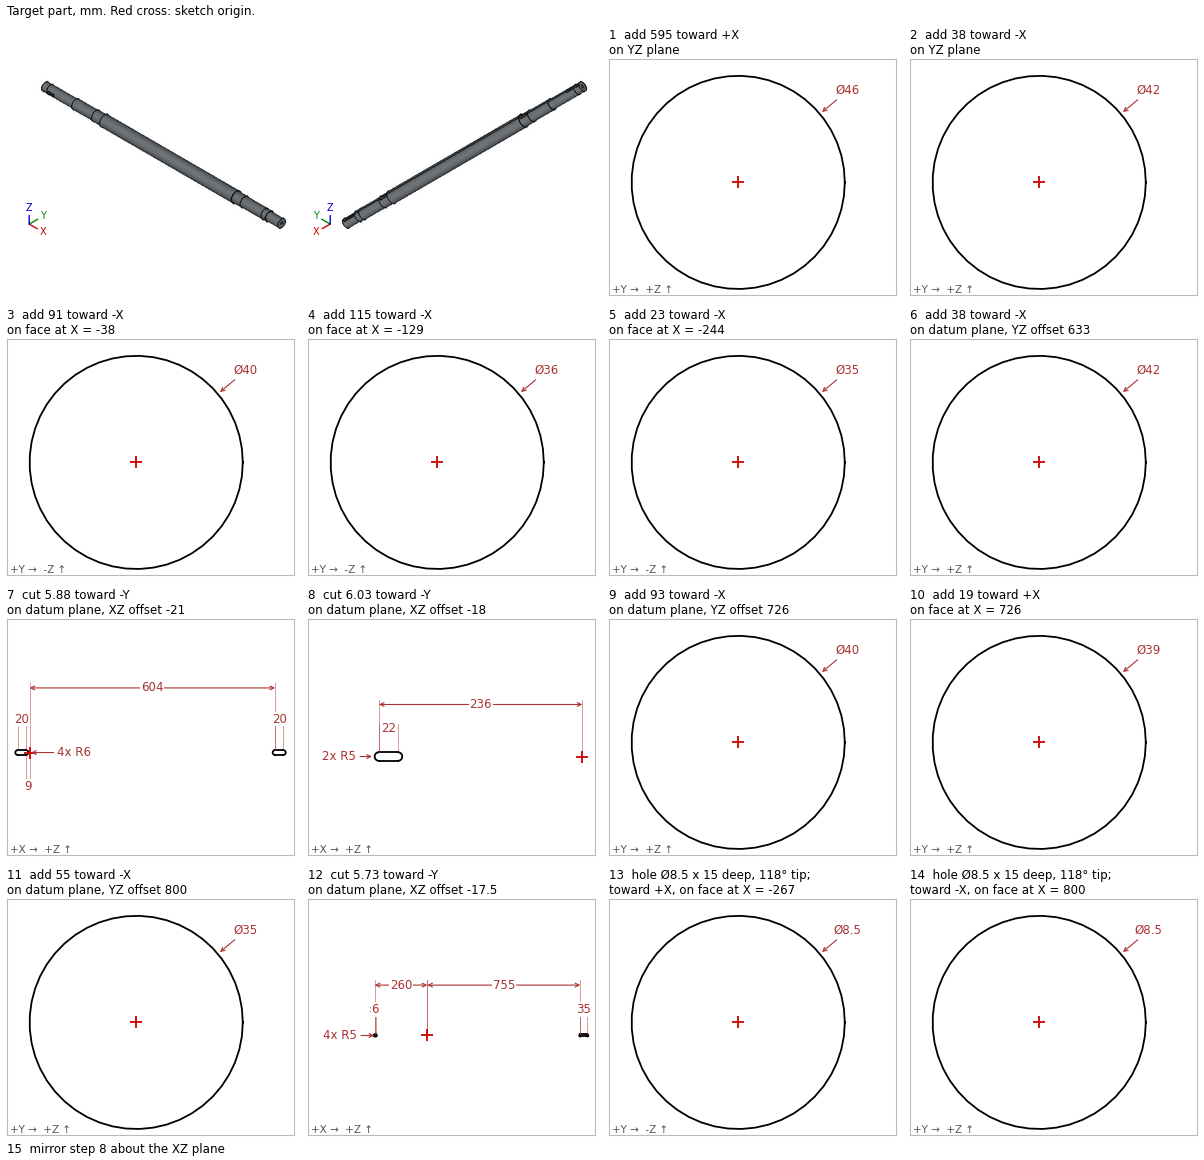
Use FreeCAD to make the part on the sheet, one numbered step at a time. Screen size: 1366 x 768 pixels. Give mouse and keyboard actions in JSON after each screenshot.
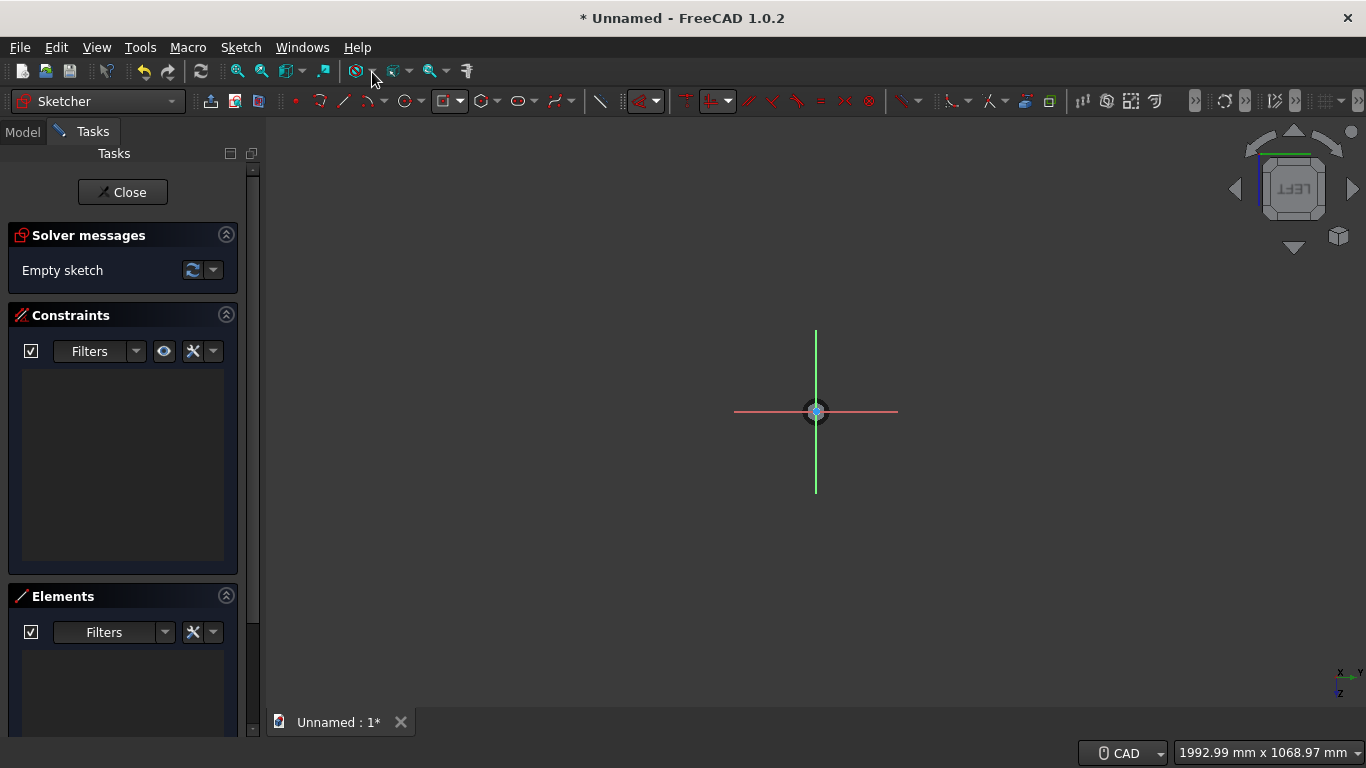
{"action": "scroll", "coordinate": [820, 412], "scroll_direction": "up", "scroll_amount": 15}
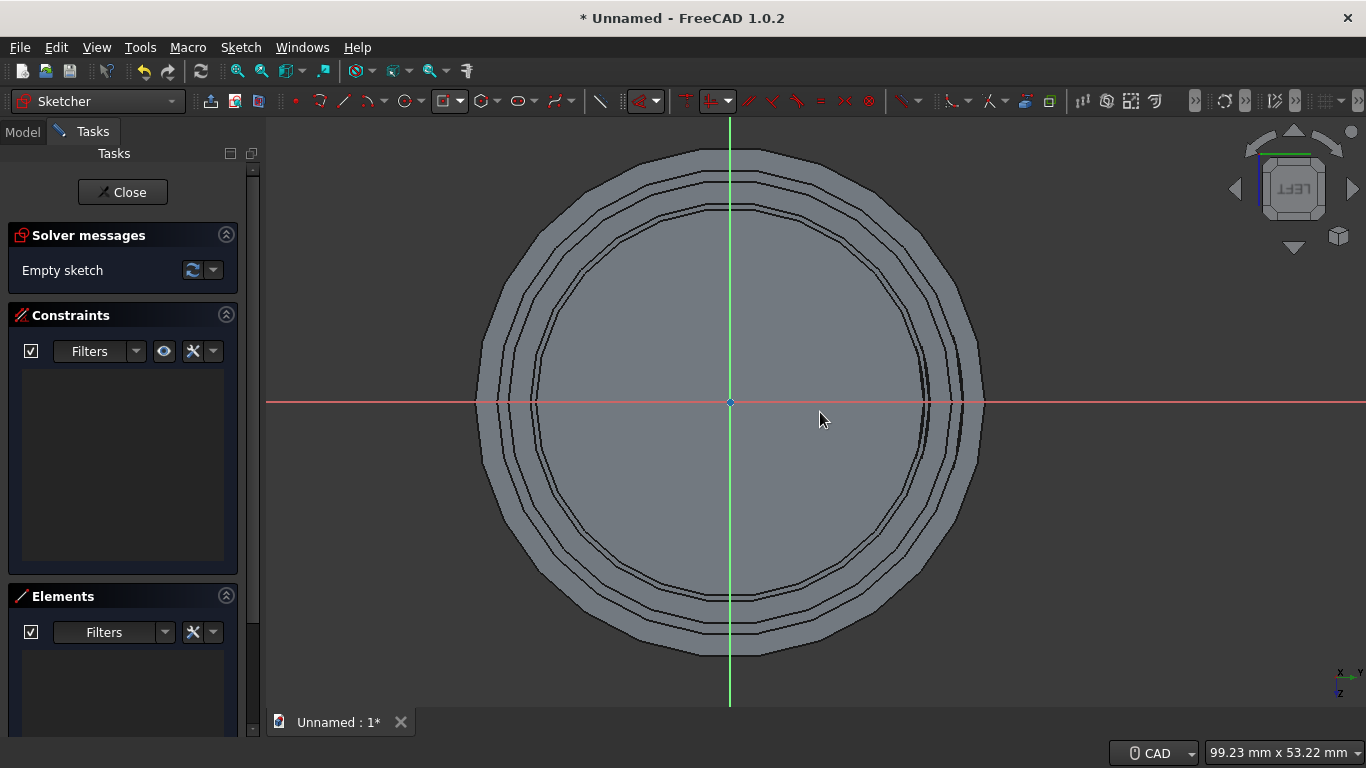
{"action": "scroll", "coordinate": [724, 399], "scroll_direction": "up", "scroll_amount": 7}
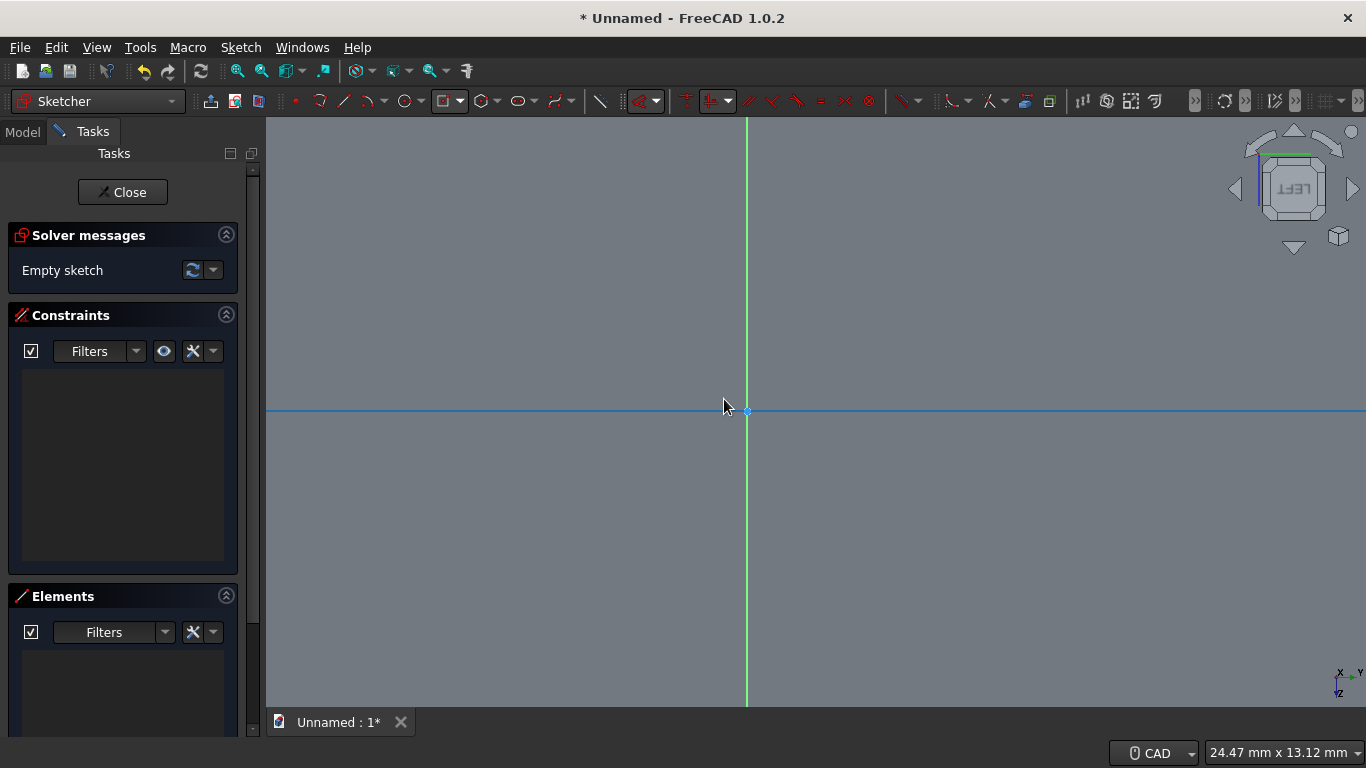
{"action": "key", "text": "g c"}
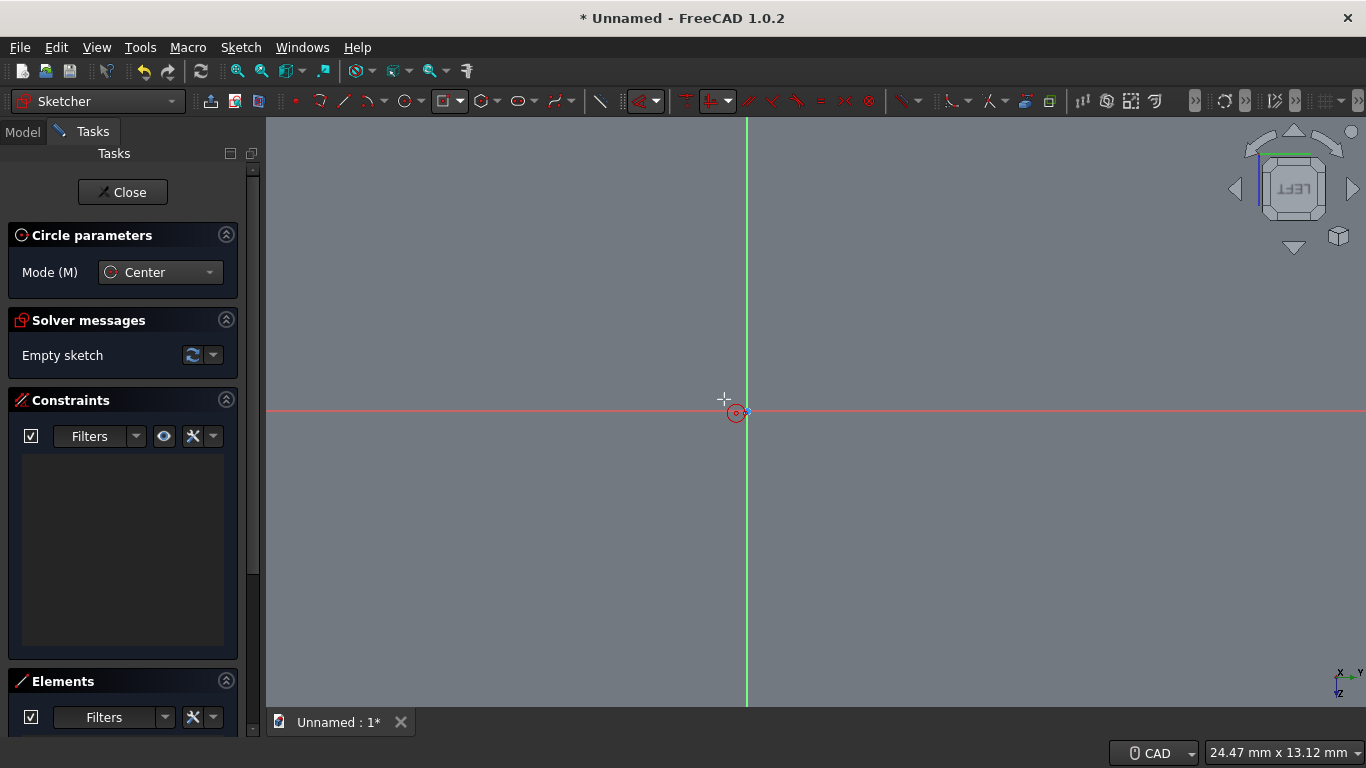
{"action": "left_click", "coordinate": [747, 411]}
{"action": "mouse_move", "coordinate": [882, 276]}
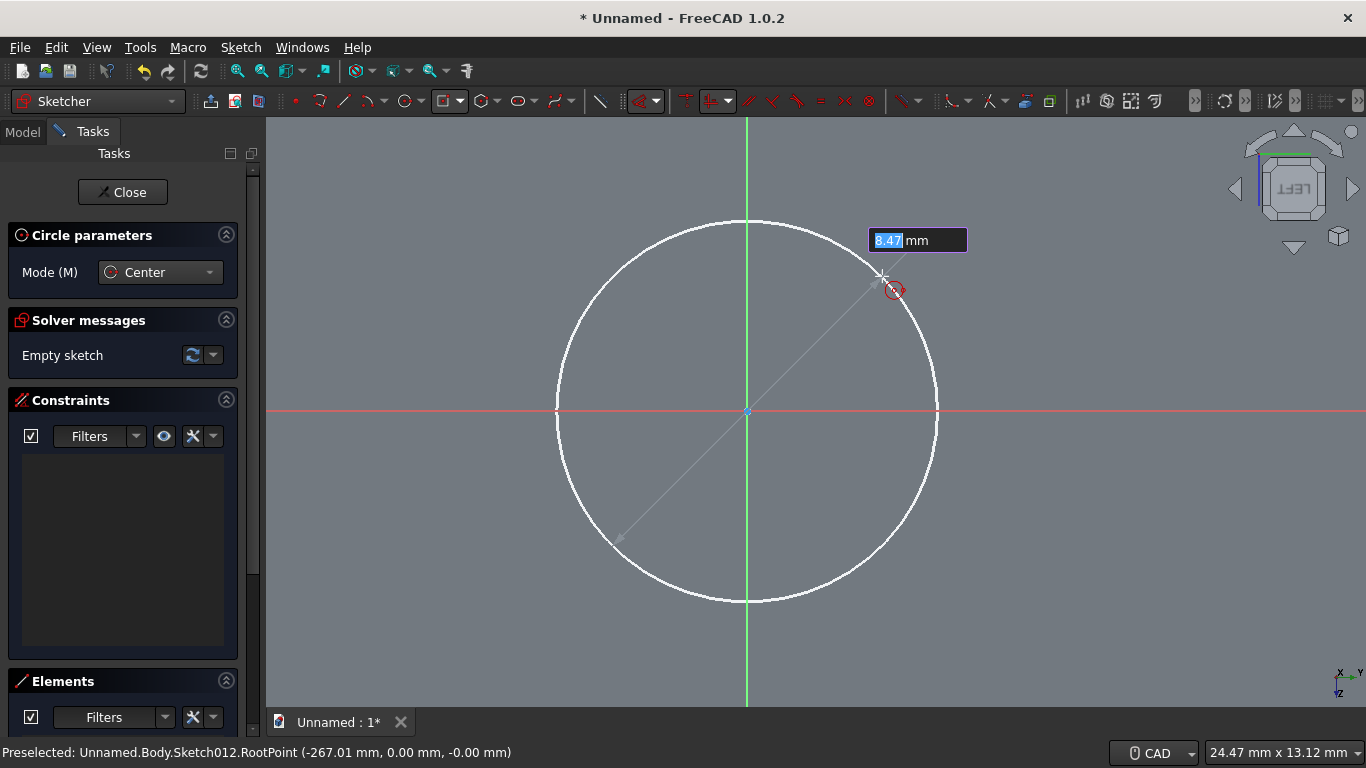
{"action": "type", "text": "8.5"}
{"action": "key", "text": "Return"}
{"action": "key", "text": "Escape"}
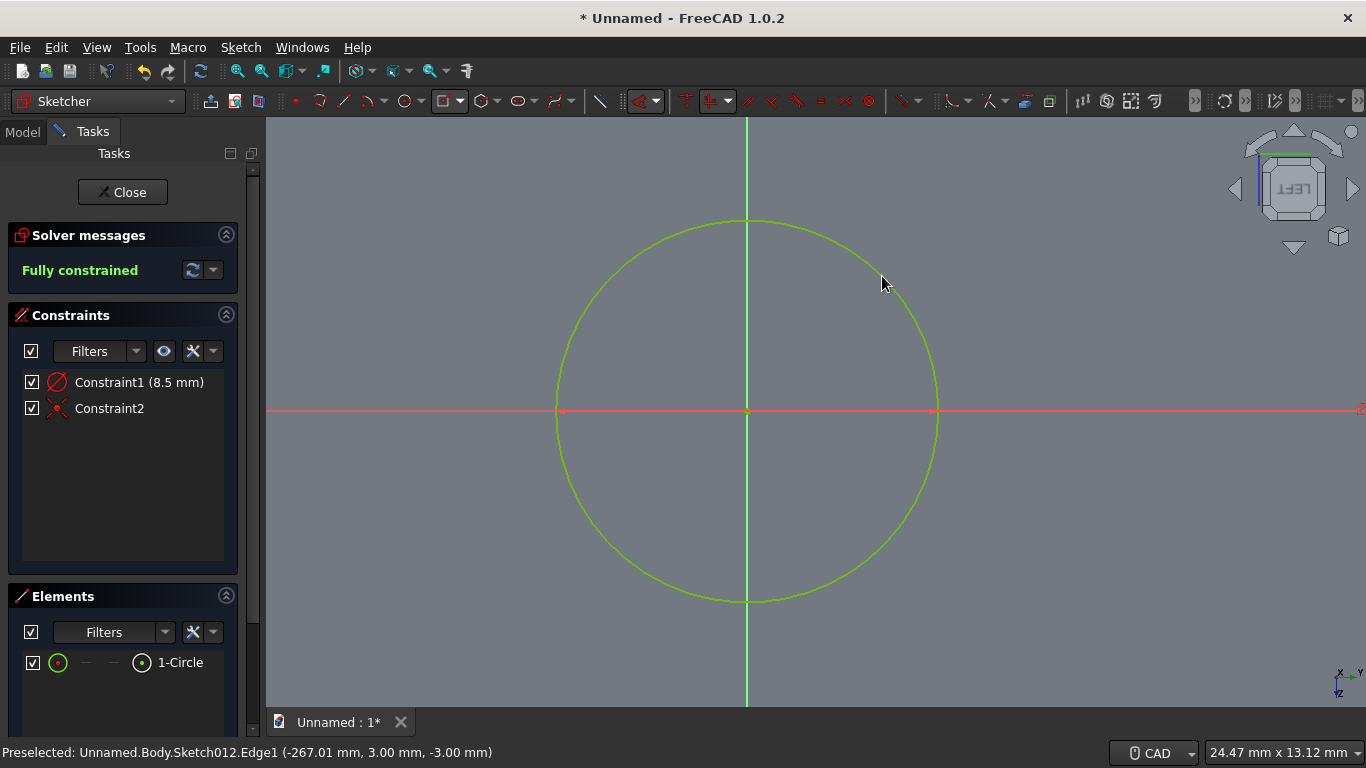
{"action": "left_click", "coordinate": [123, 192]}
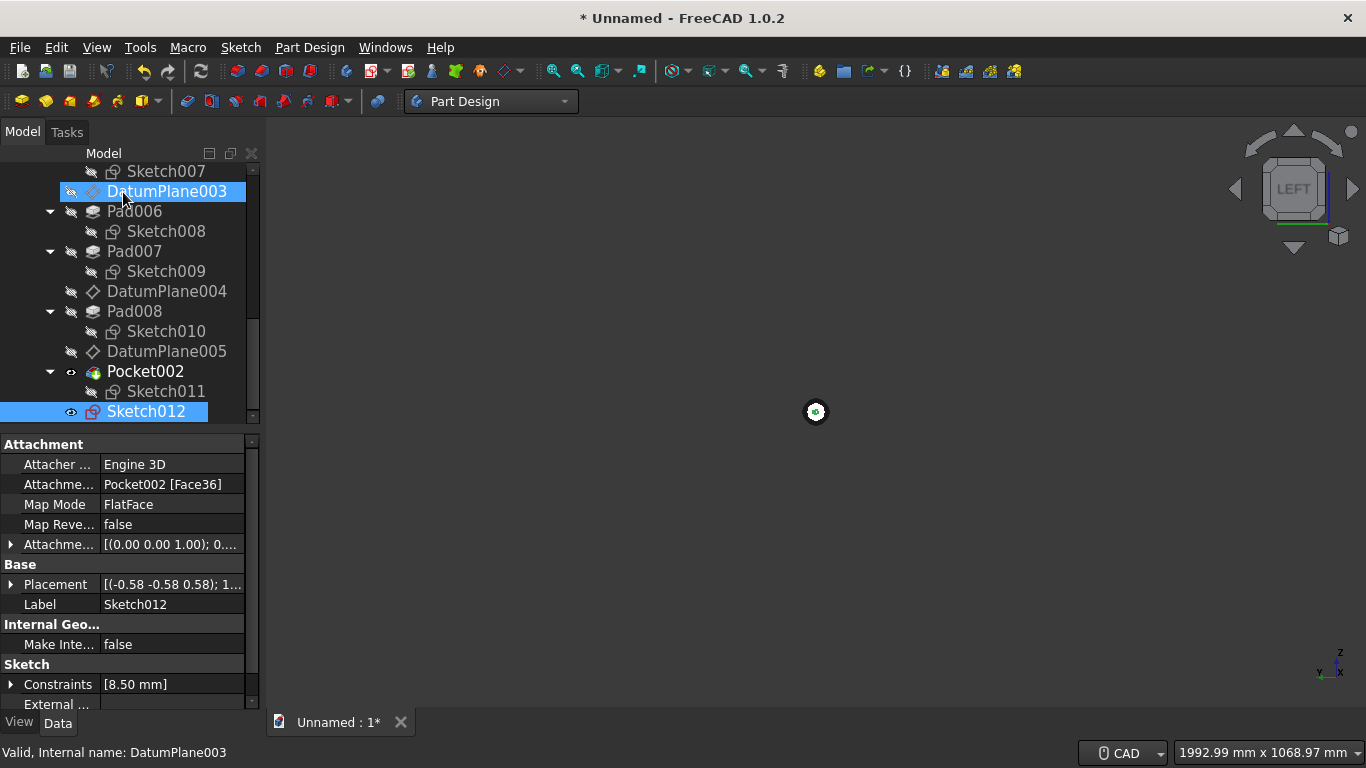
{"action": "left_click", "coordinate": [212, 102]}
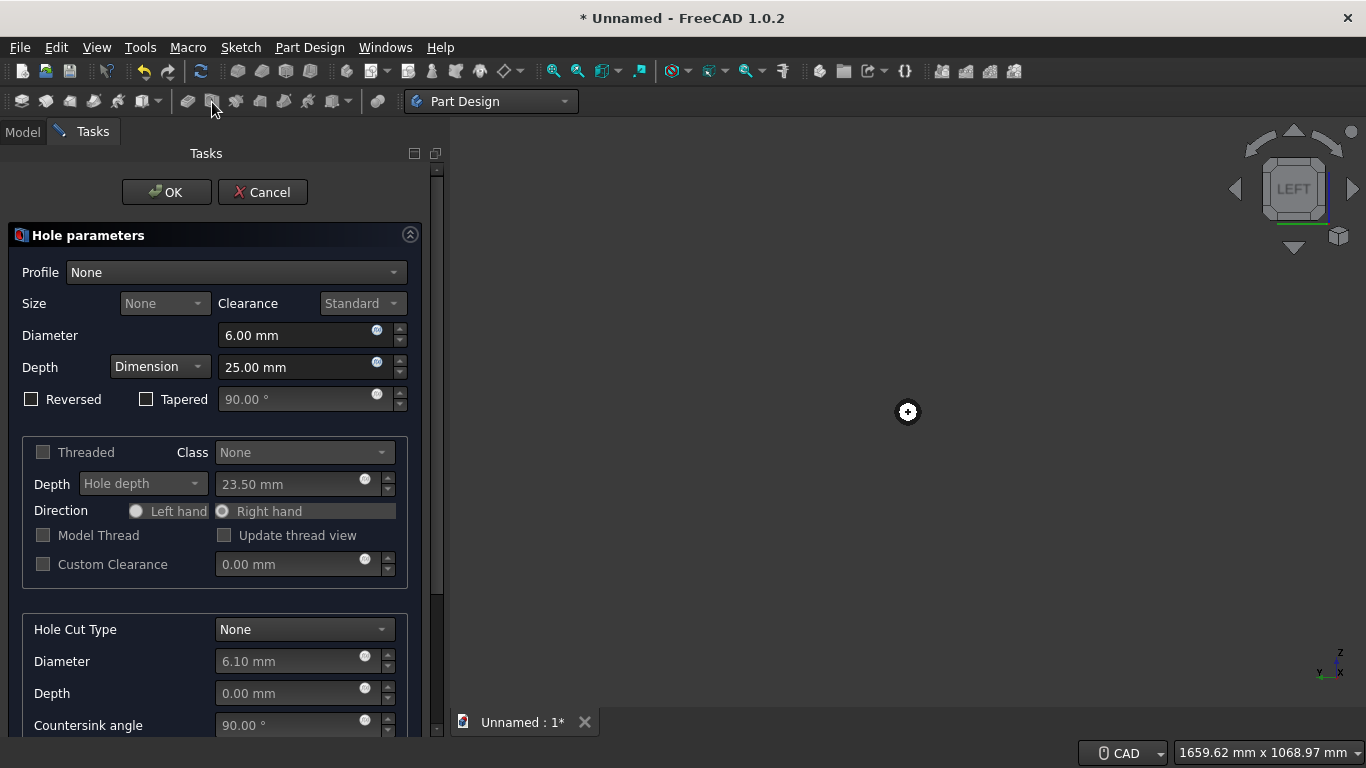
{"action": "triple_click", "coordinate": [305, 335]}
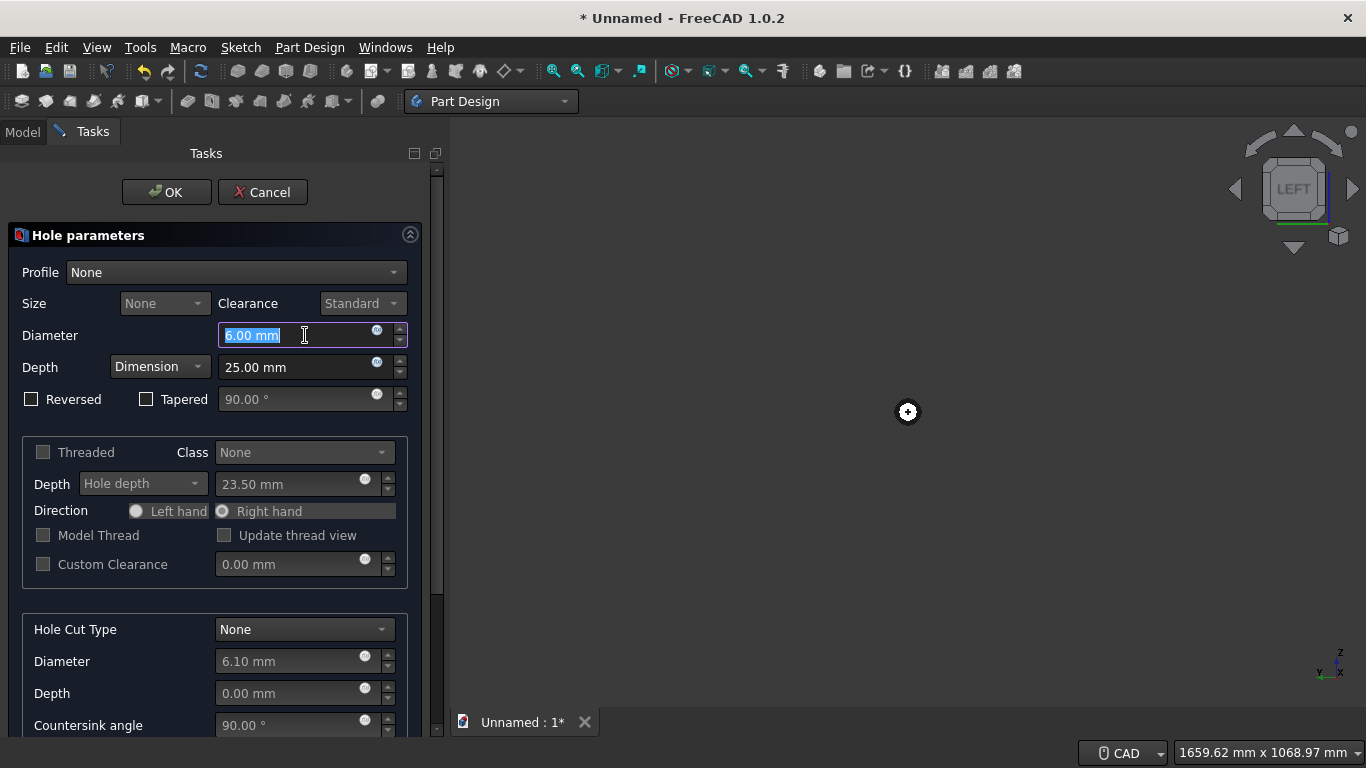
{"action": "type", "text": "8.5"}
{"action": "key", "text": "Tab"}